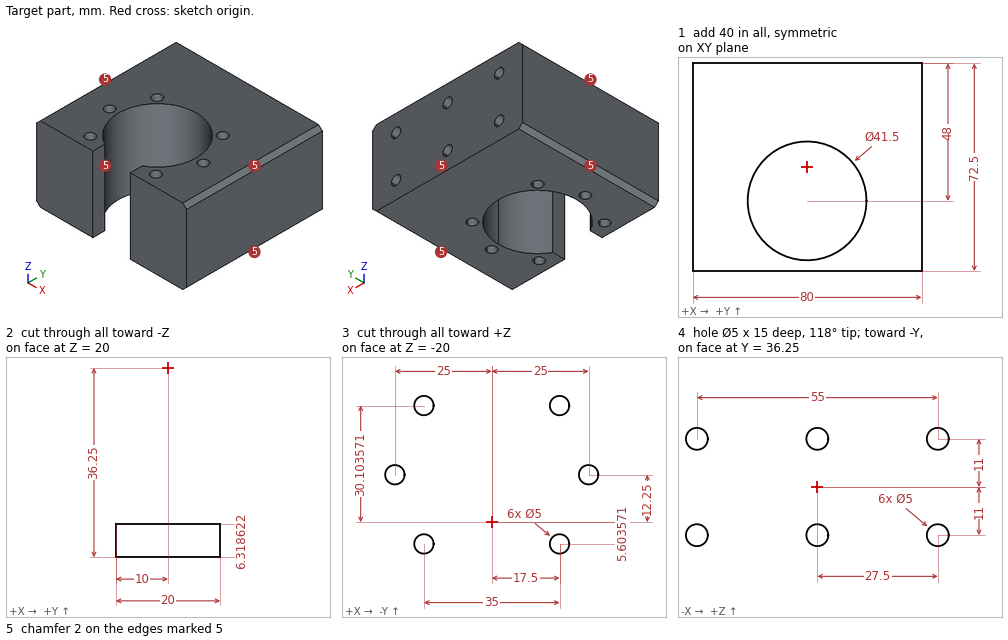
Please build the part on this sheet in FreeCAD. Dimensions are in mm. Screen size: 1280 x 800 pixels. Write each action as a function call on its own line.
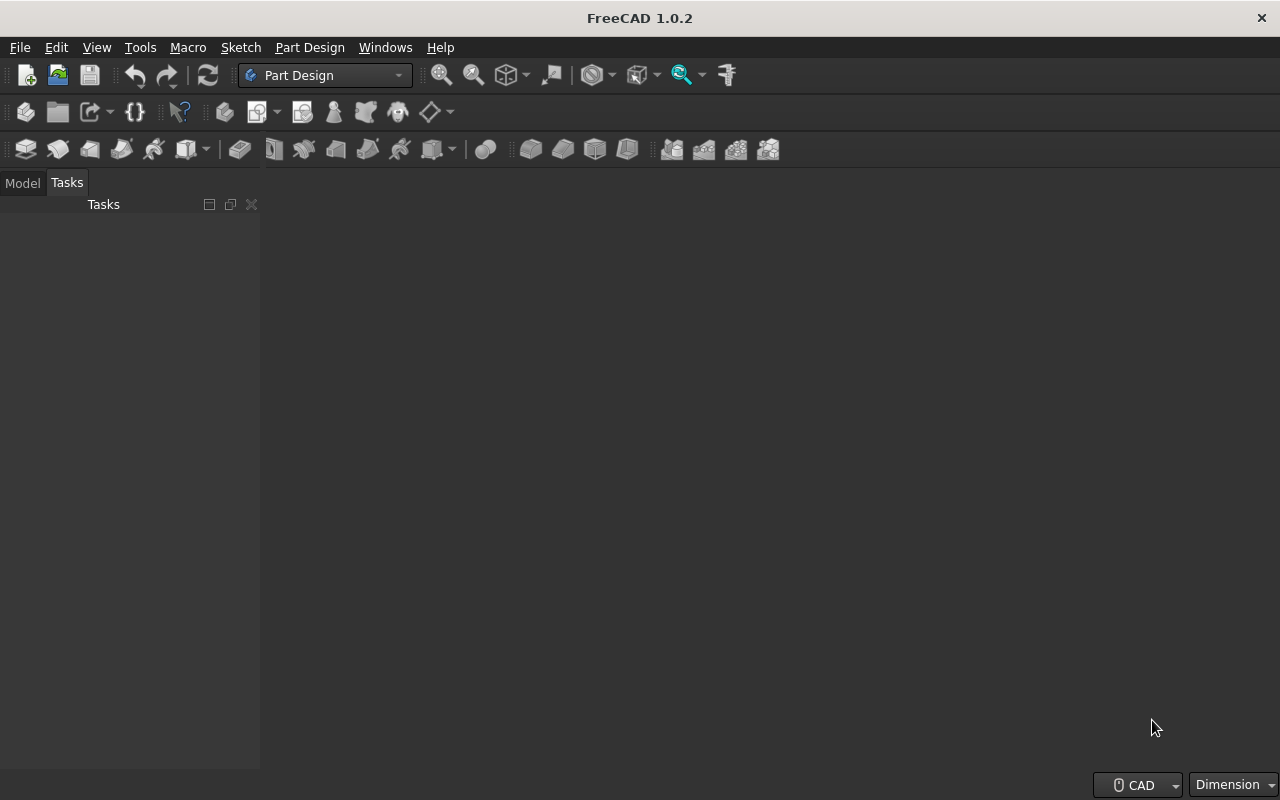
key(ctrl+n)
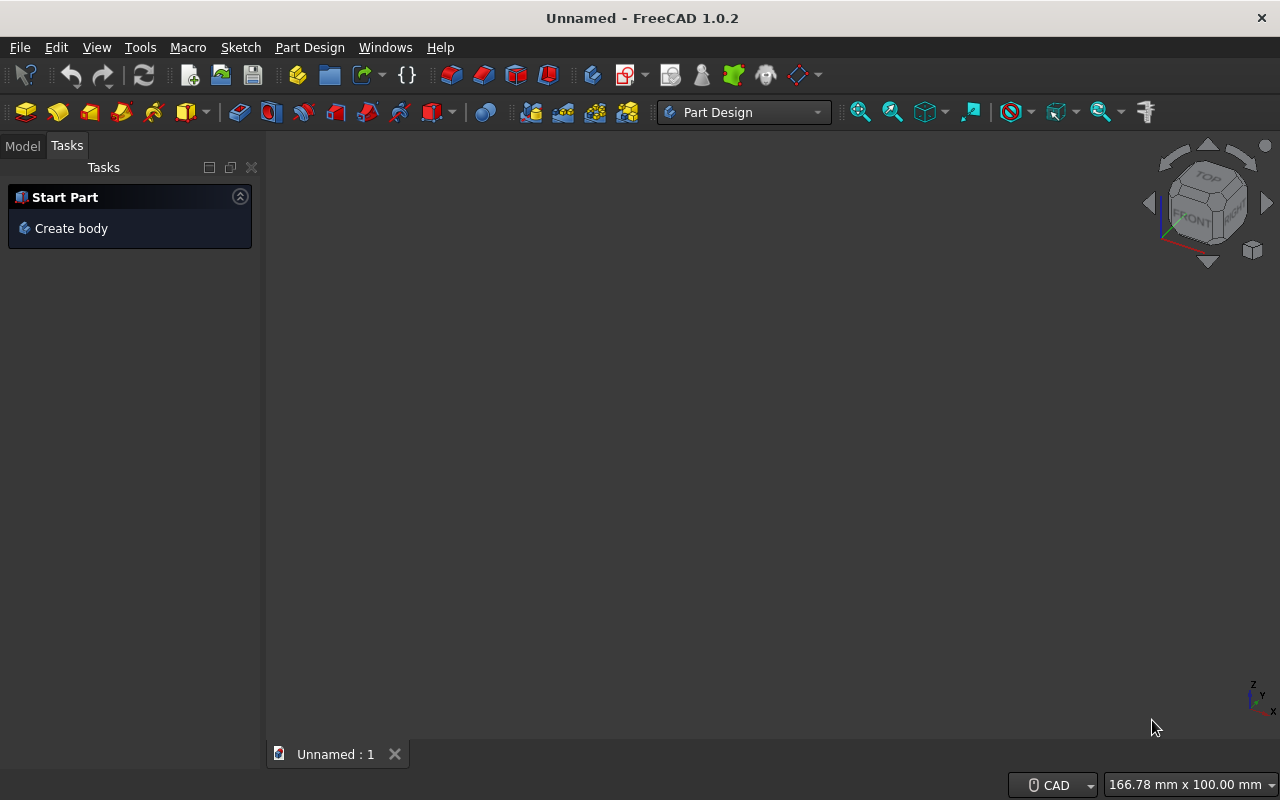
click(626, 76)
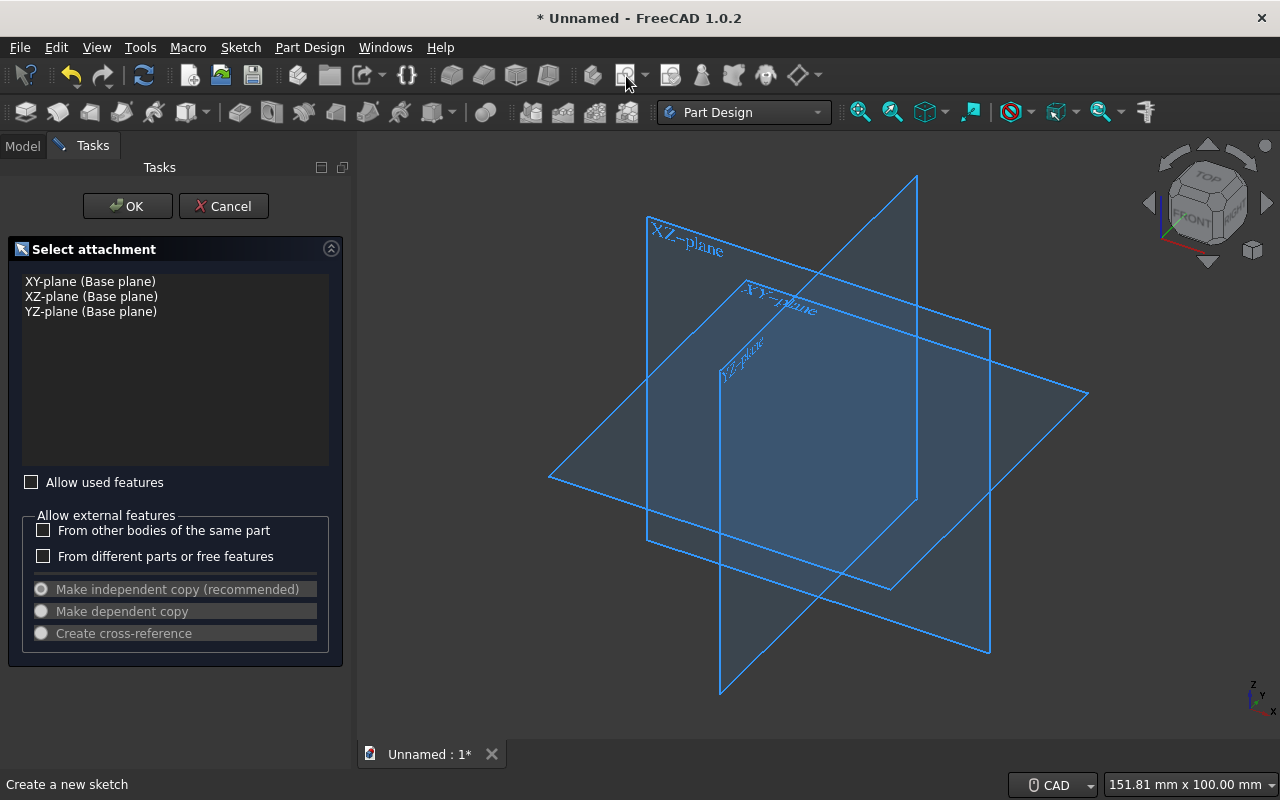
click(82, 282)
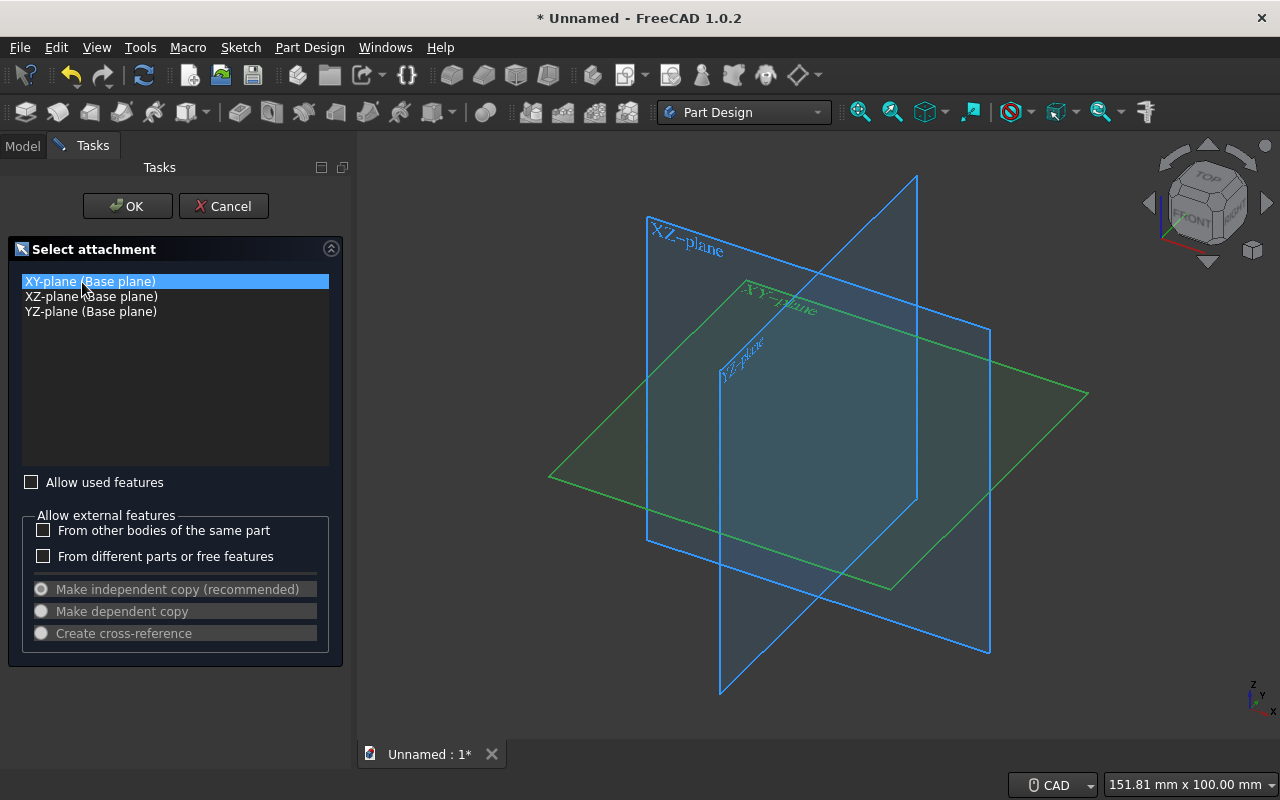
click(128, 206)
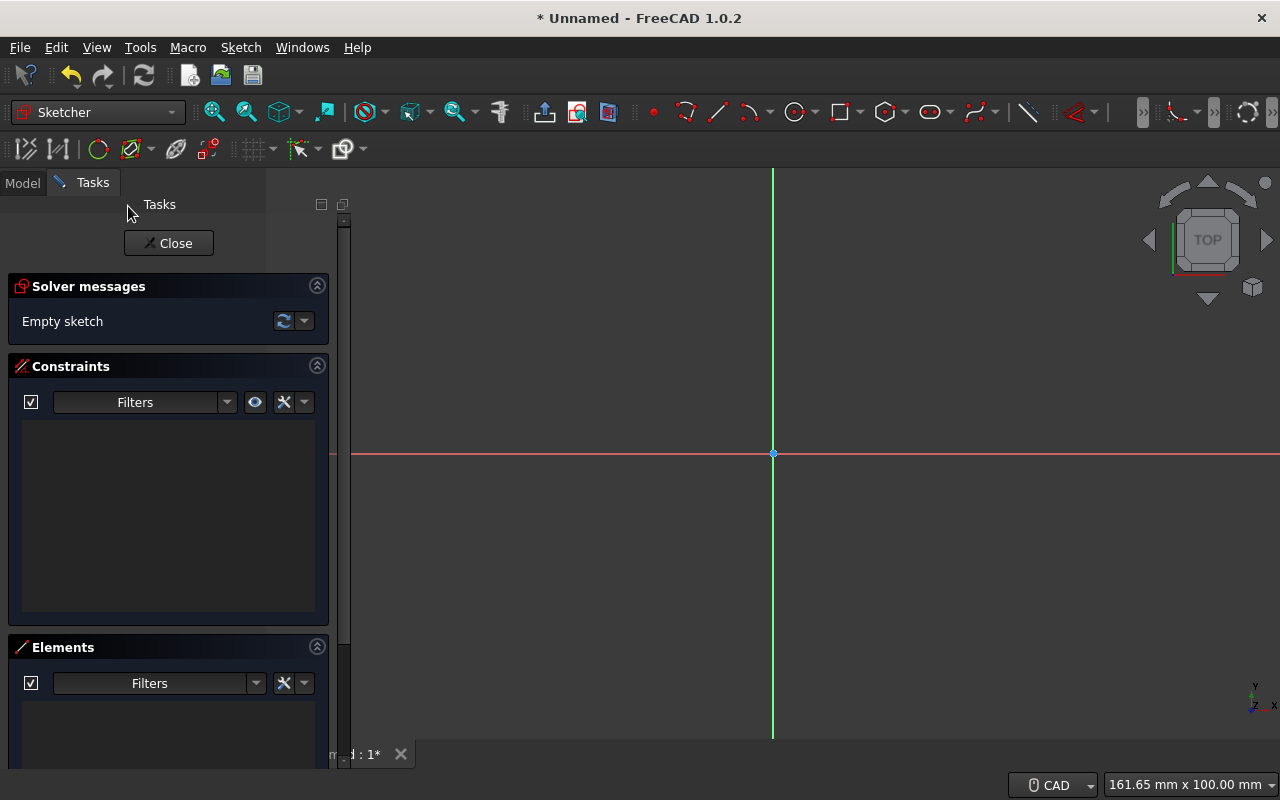
key(g)
key(v)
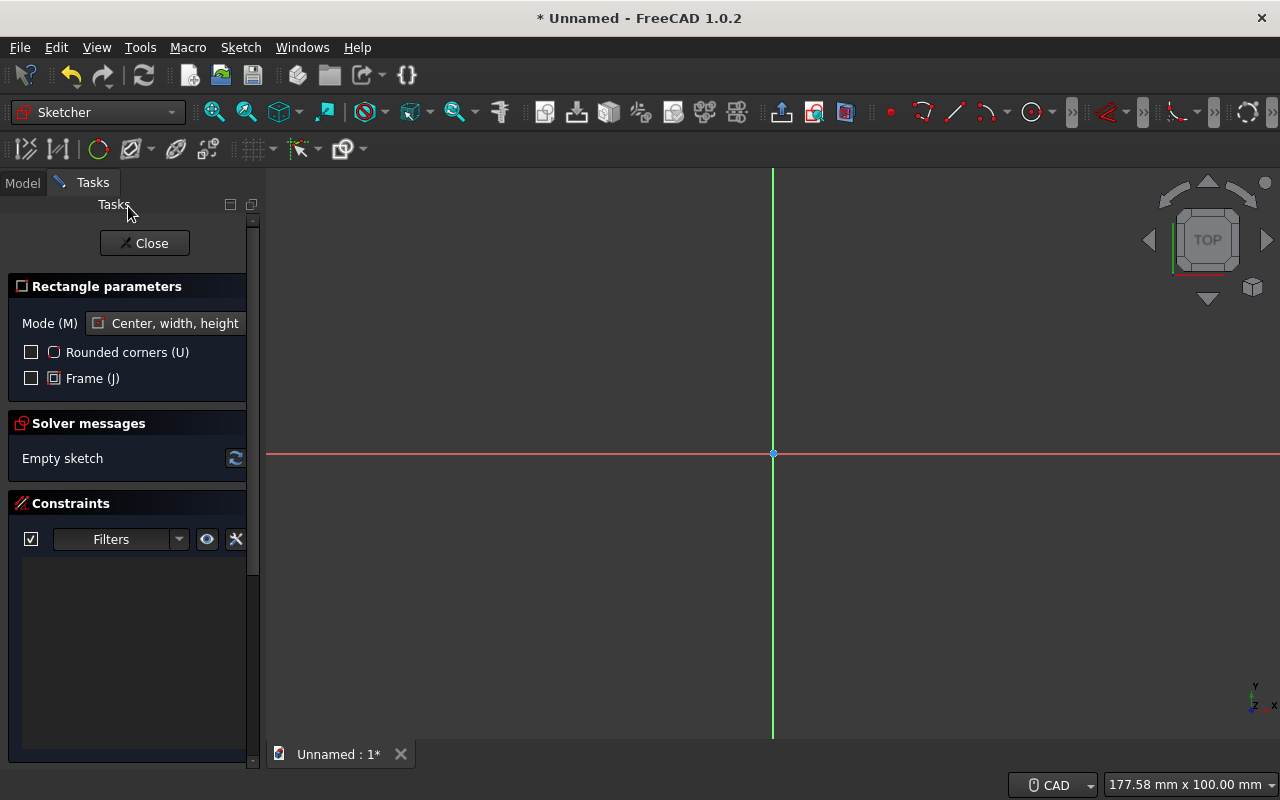
click(773, 454)
move(1001, 247)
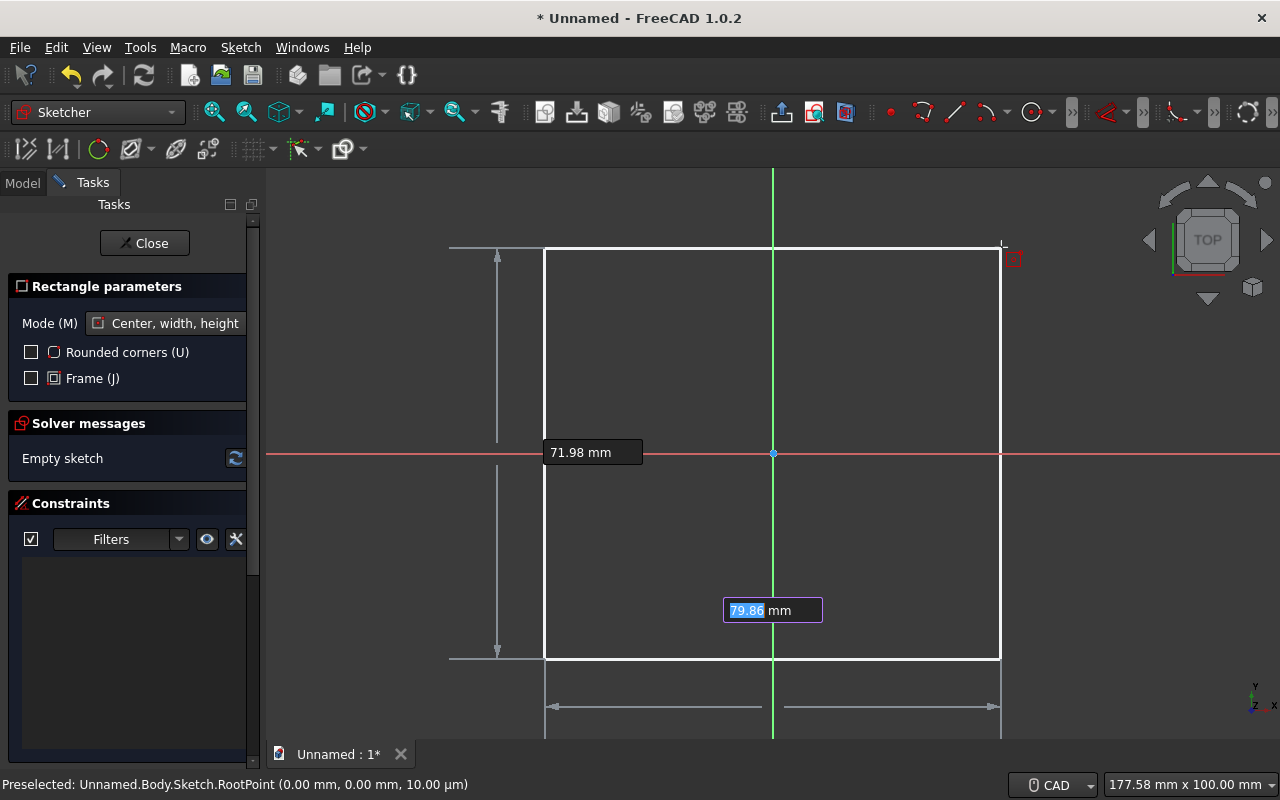
text(80)
key(Tab)
text(72.5)
key(Return)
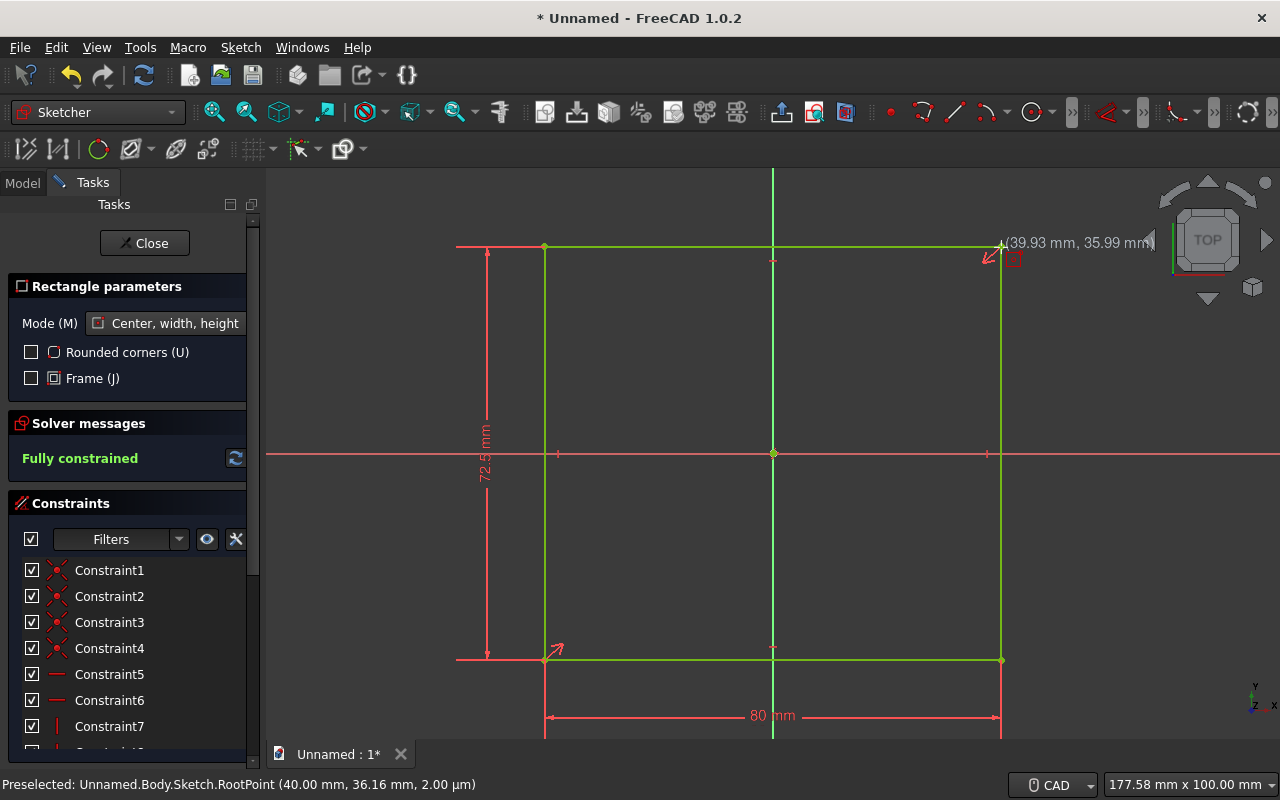
key(g)
key(c)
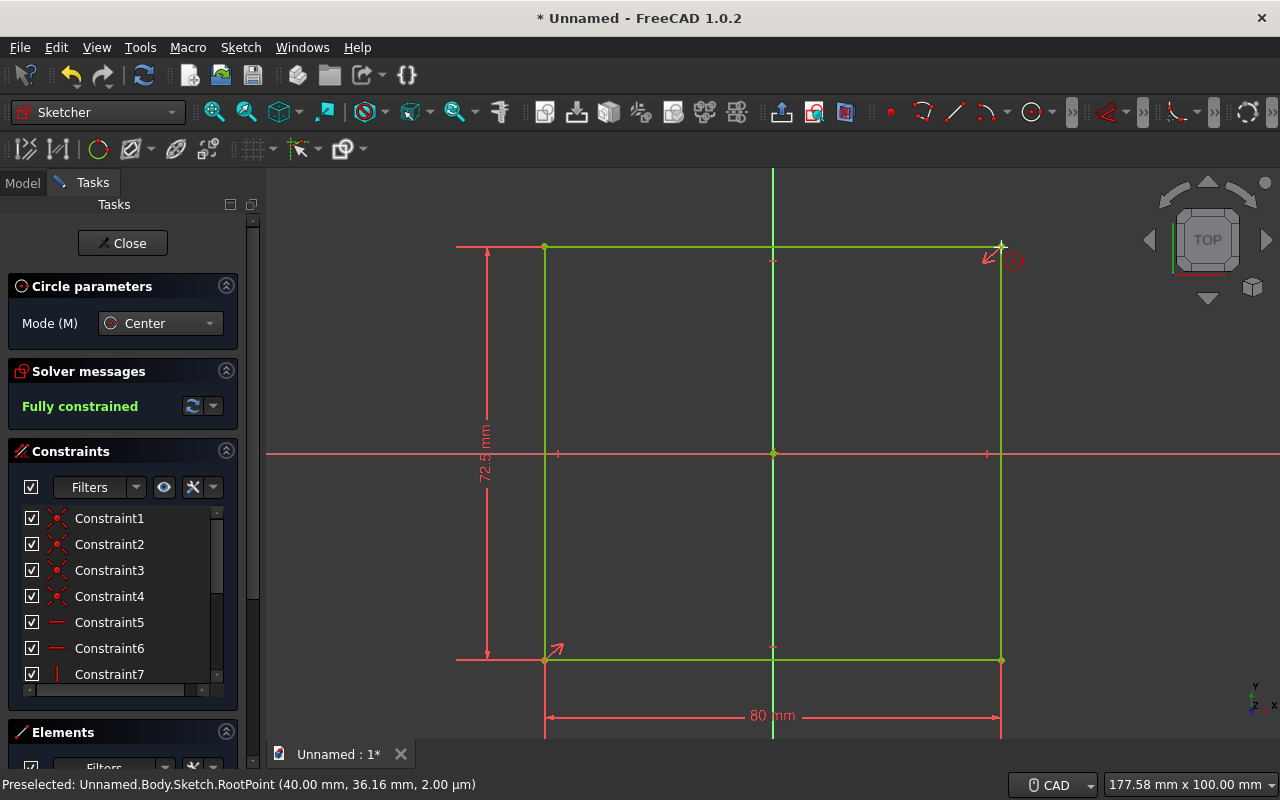
click(773, 521)
move(857, 437)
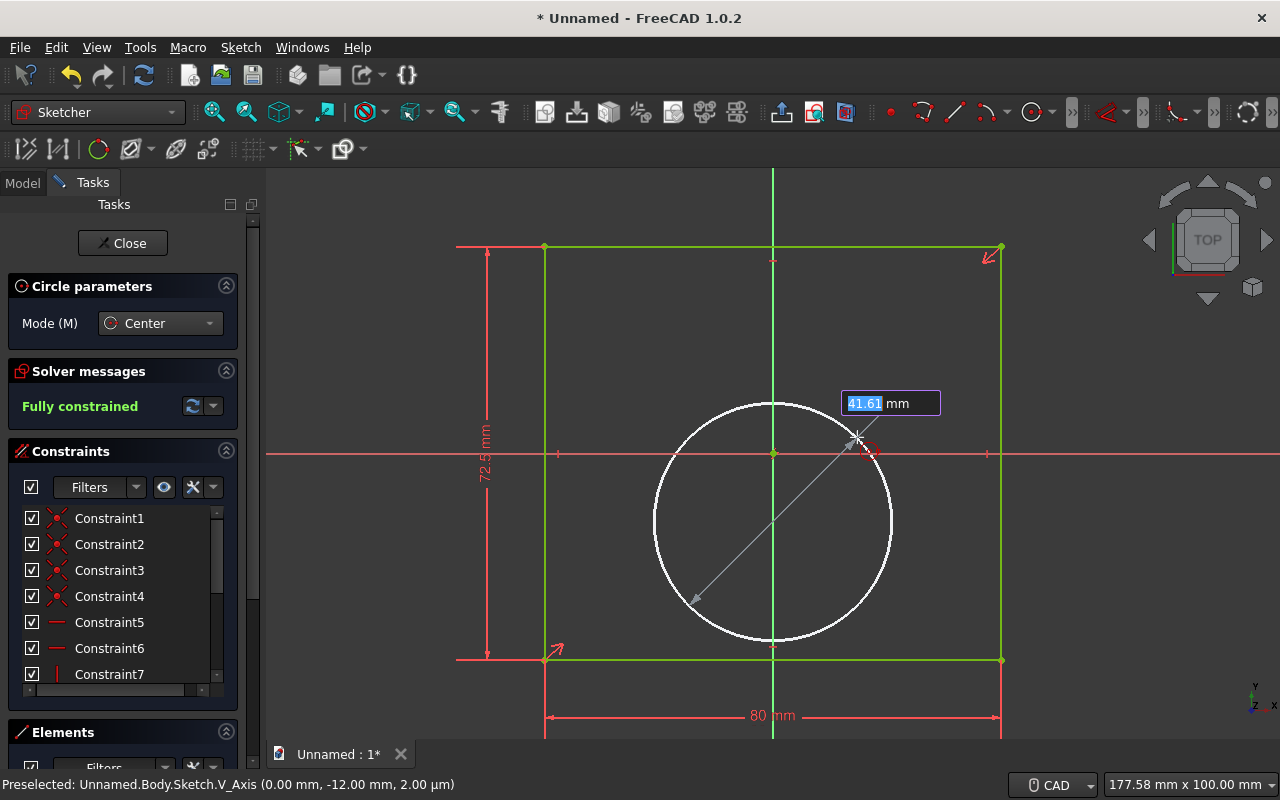
text(41.5)
key(Return)
key(Escape)